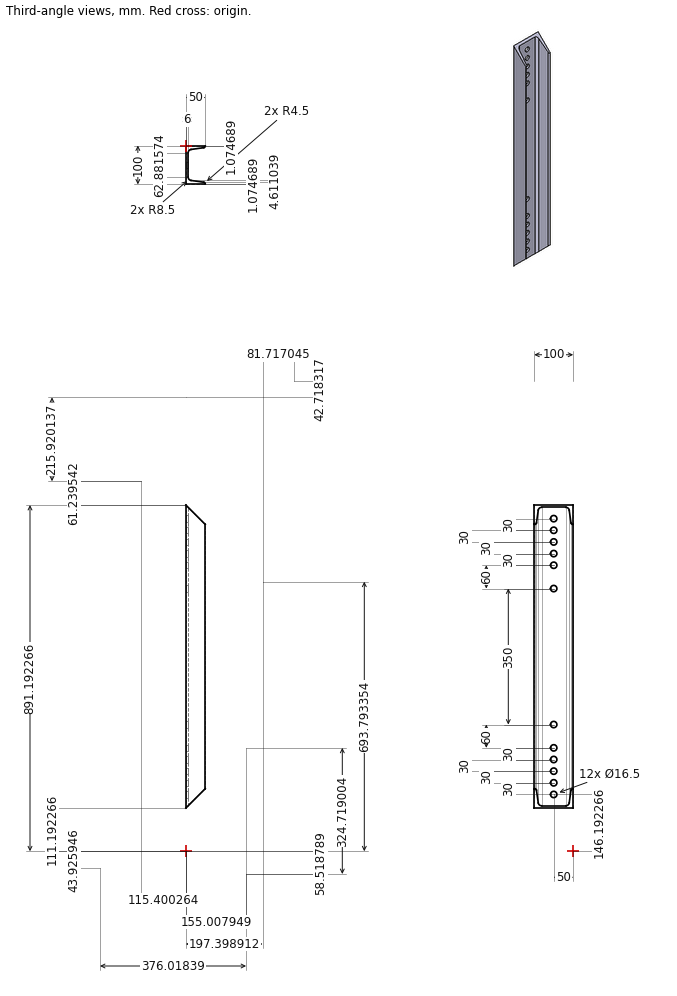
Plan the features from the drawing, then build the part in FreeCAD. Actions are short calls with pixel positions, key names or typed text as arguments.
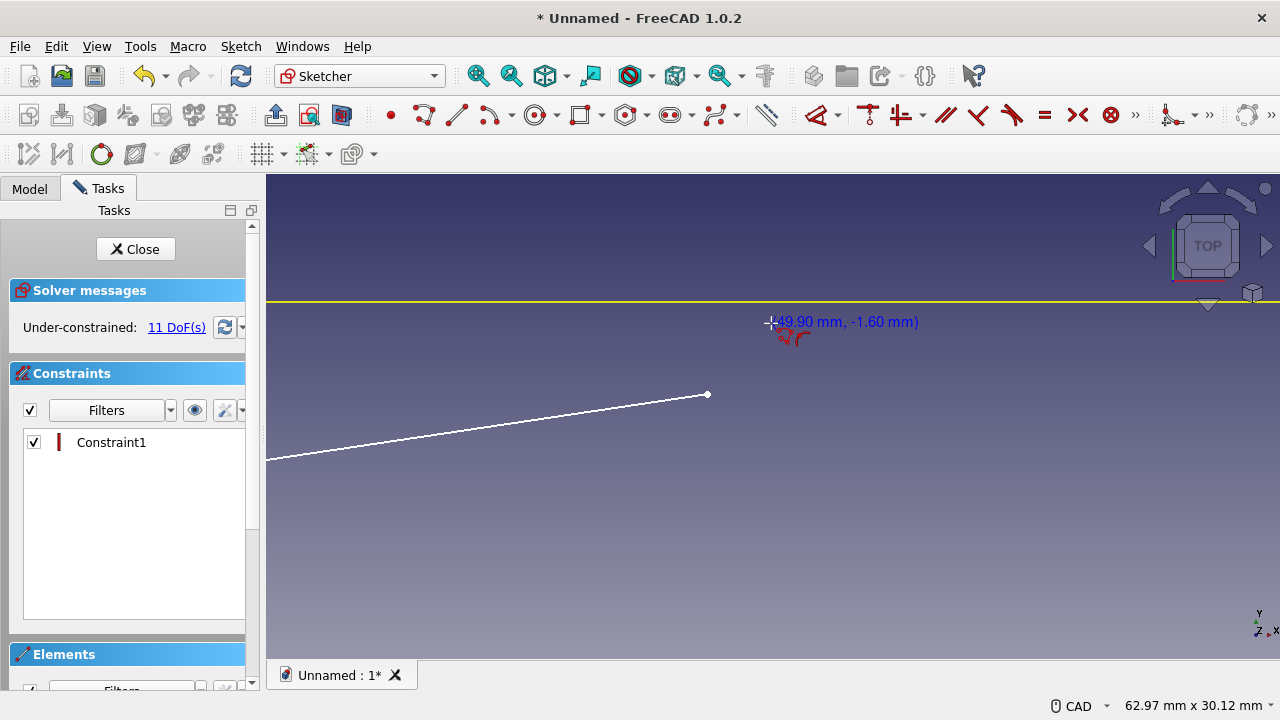
click(770, 319)
click(770, 302)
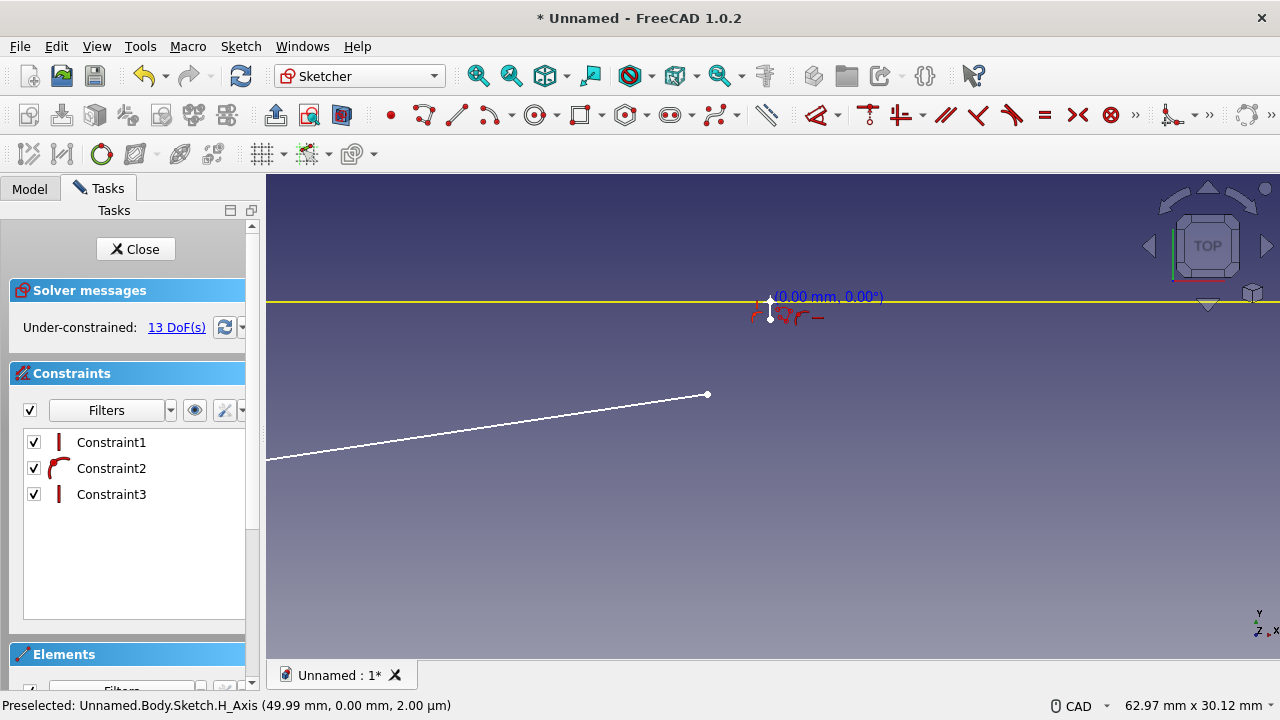
scroll(790, 242, down, 8)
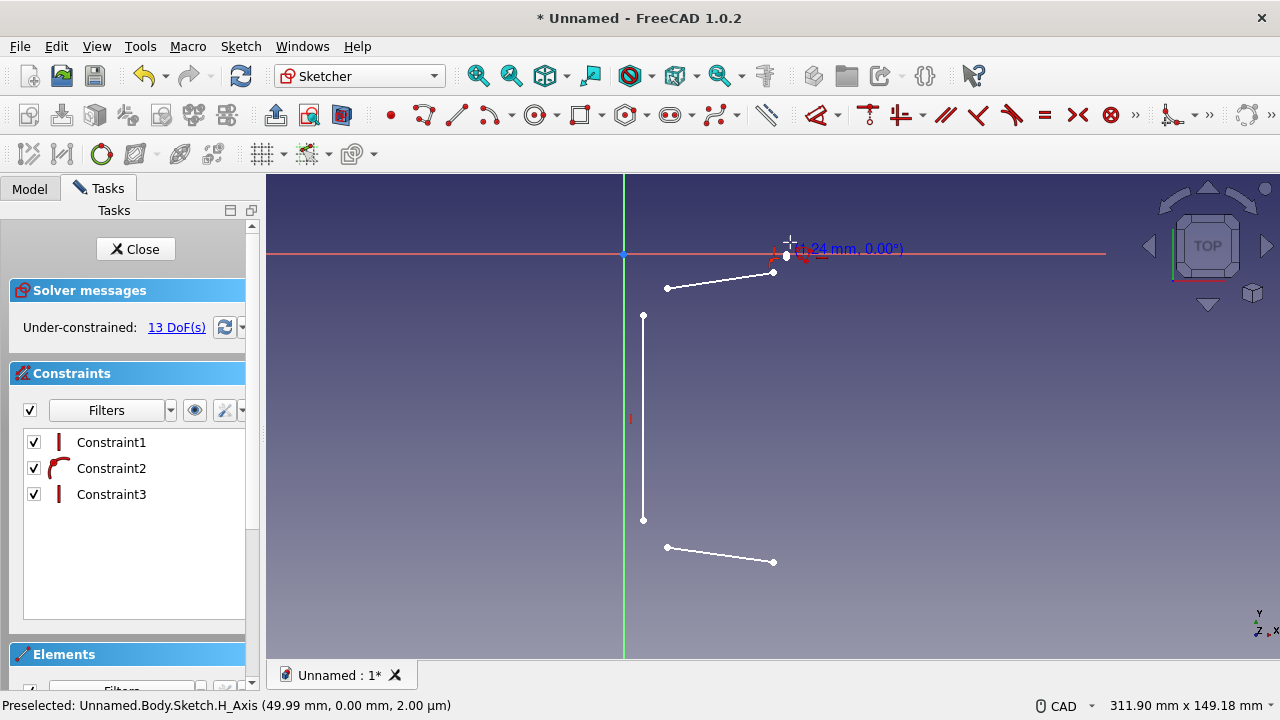
click(624, 254)
click(633, 579)
click(786, 579)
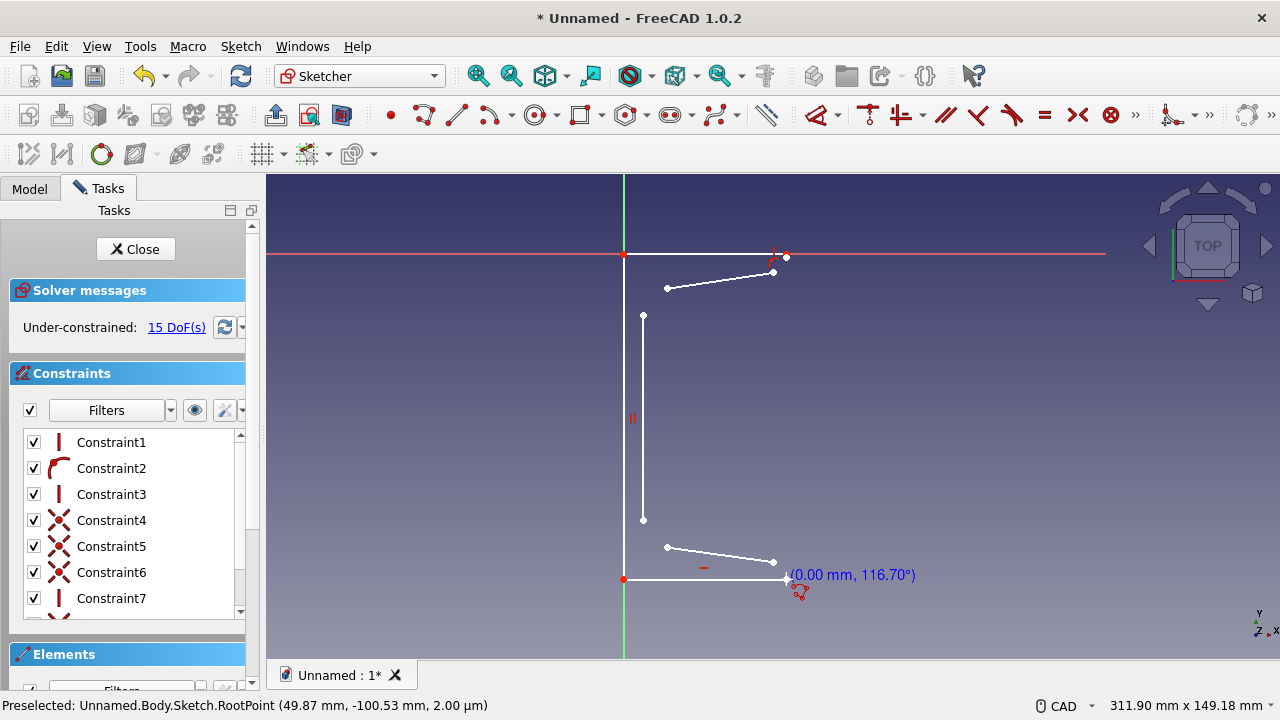
scroll(786, 576, up, 8)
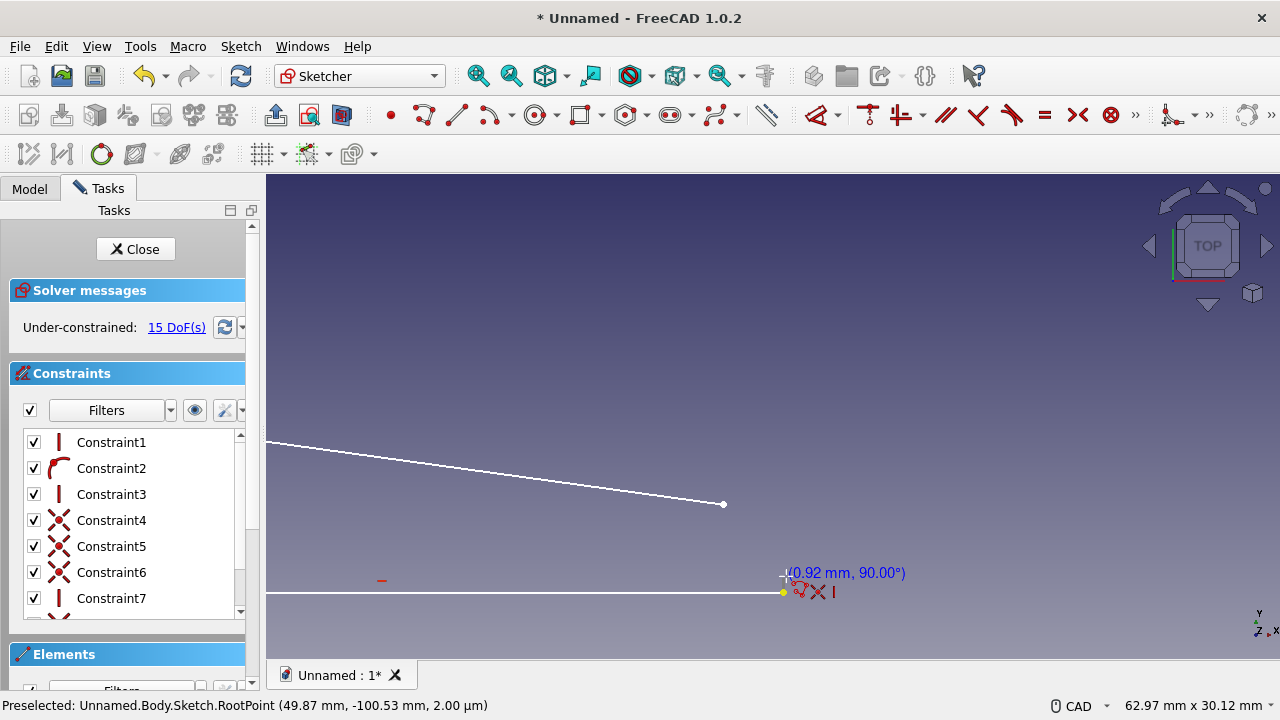
click(784, 572)
right_click(784, 572)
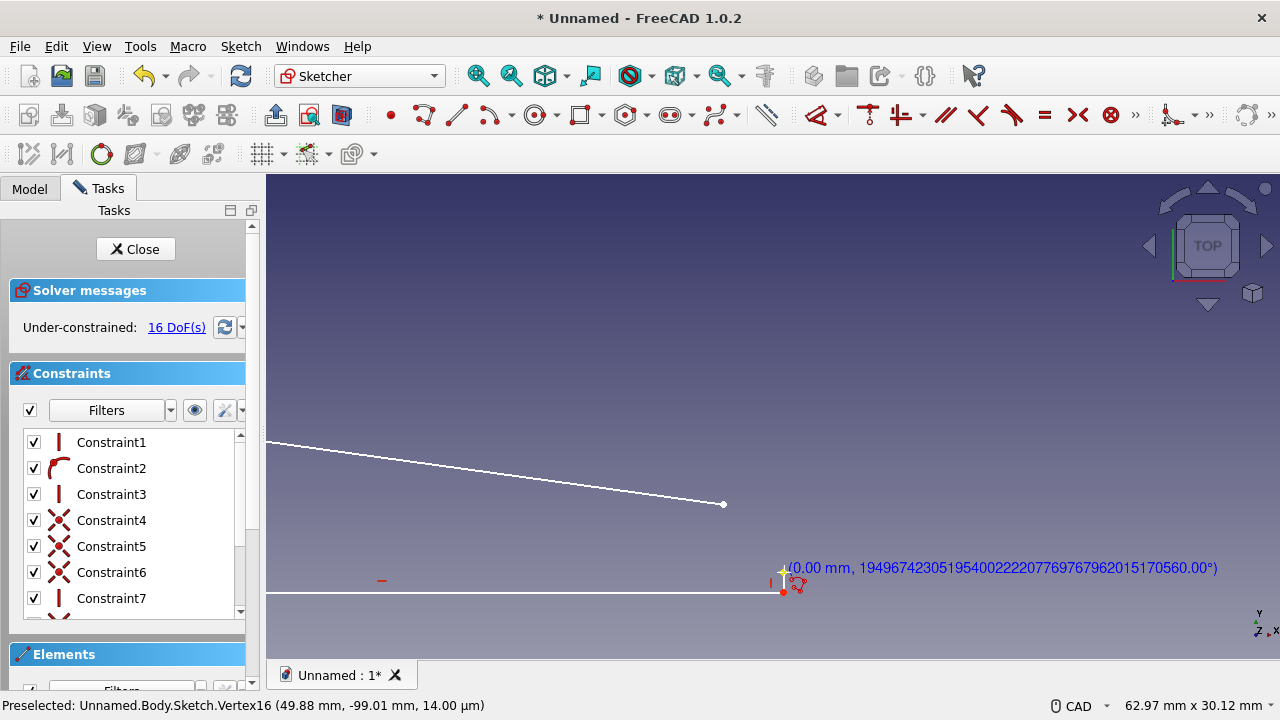
click(512, 116)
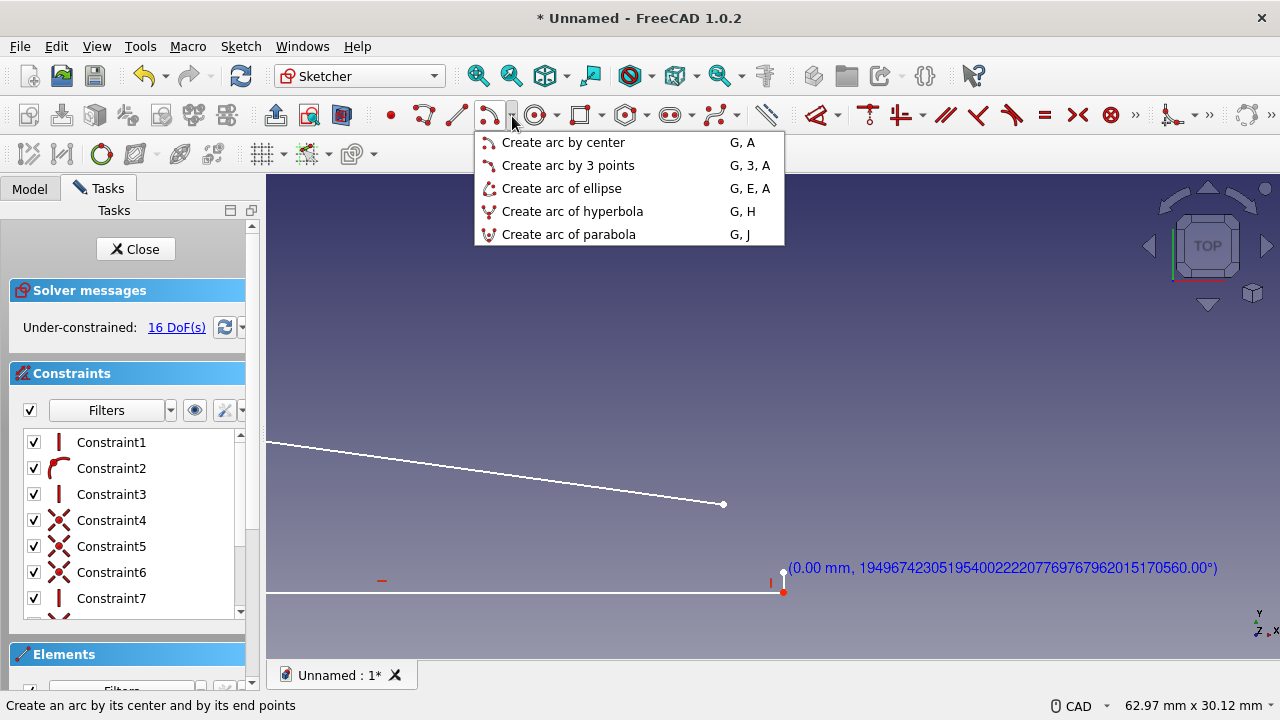
click(630, 166)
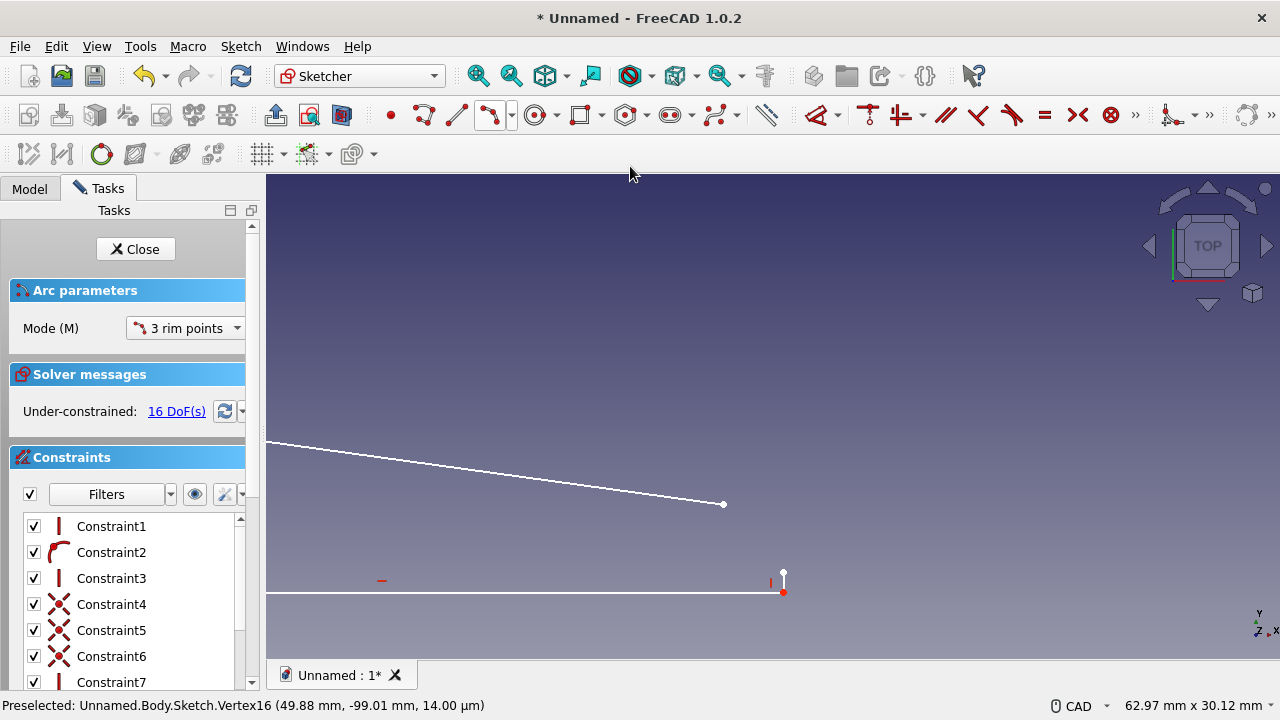
scroll(786, 577, down, 8)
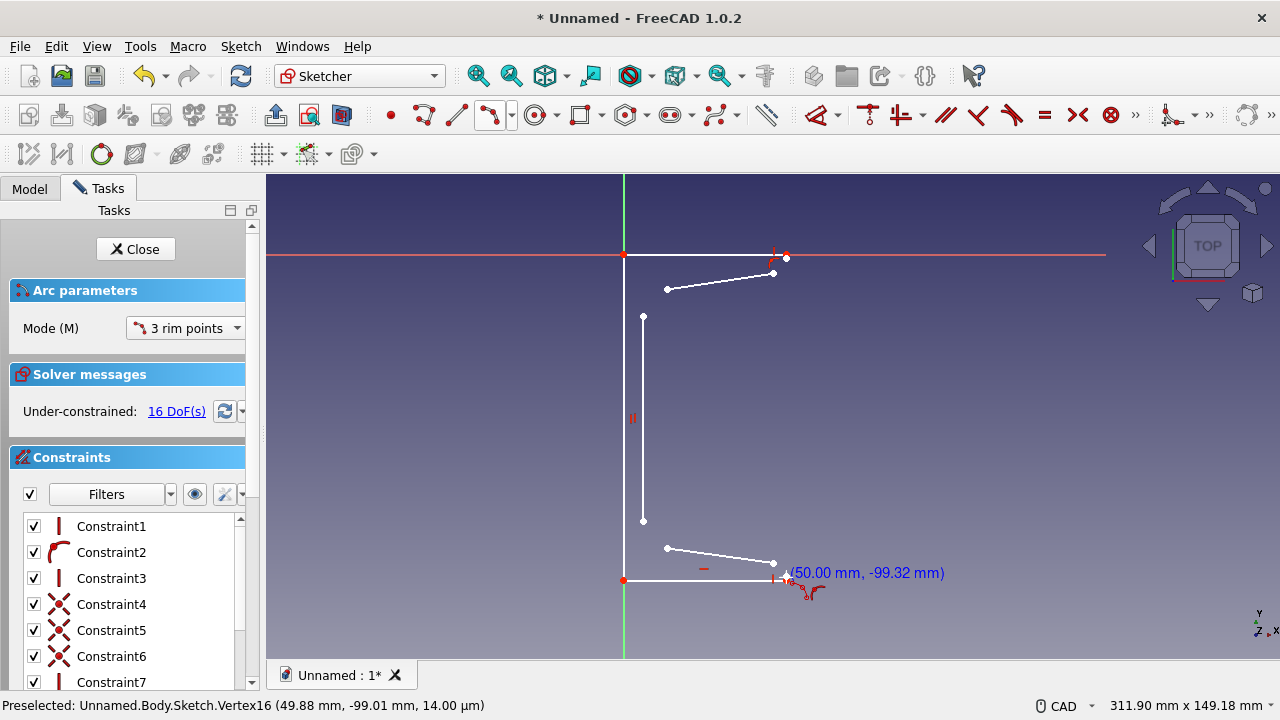
click(668, 548)
click(643, 522)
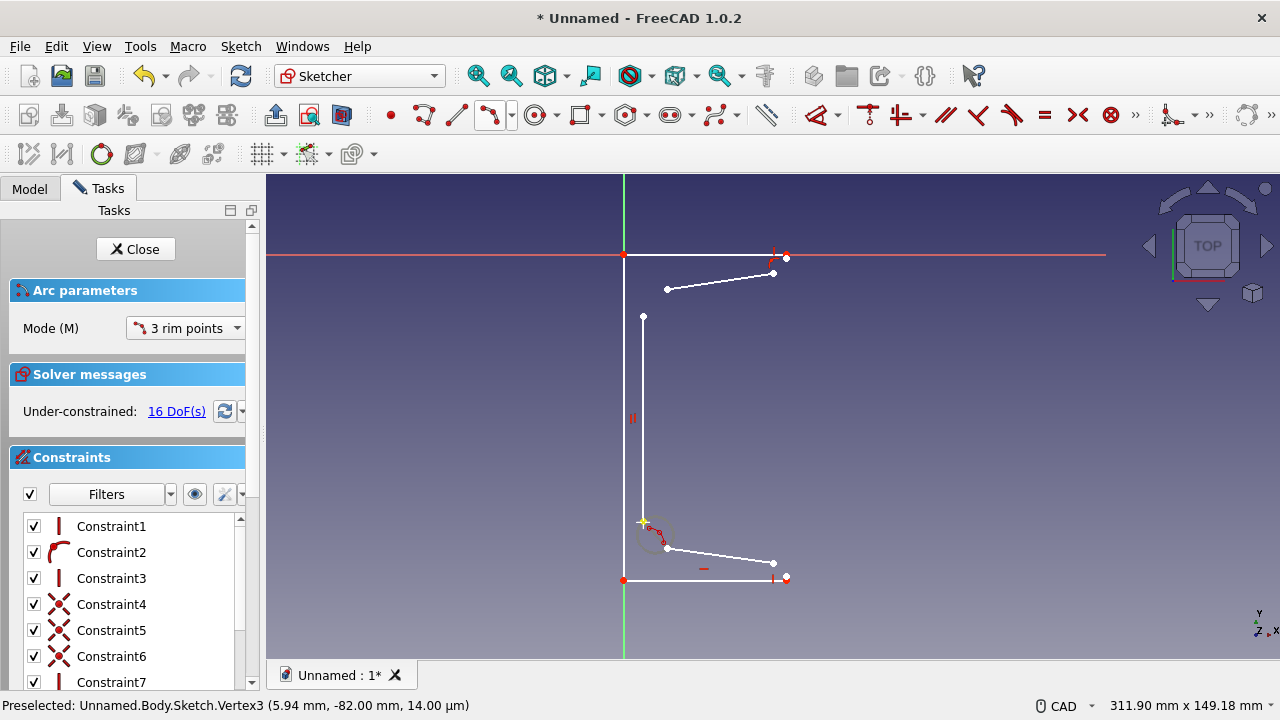
scroll(650, 538, up, 5)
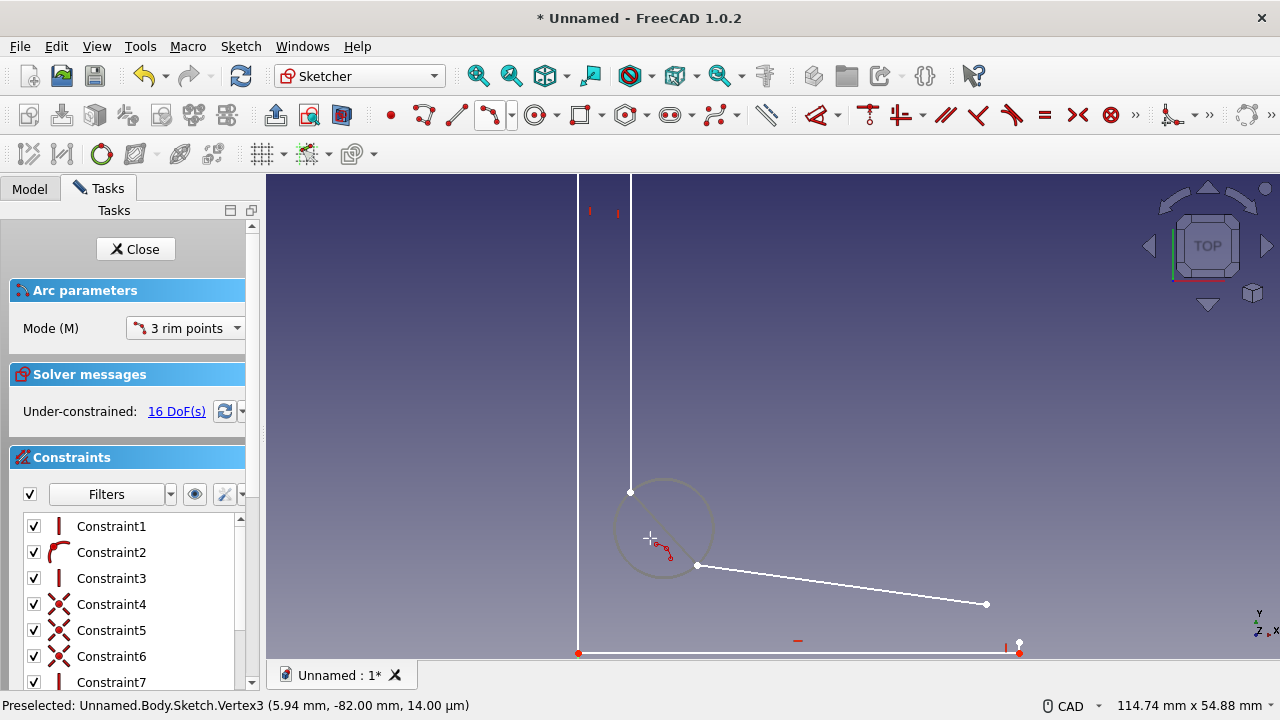
click(650, 536)